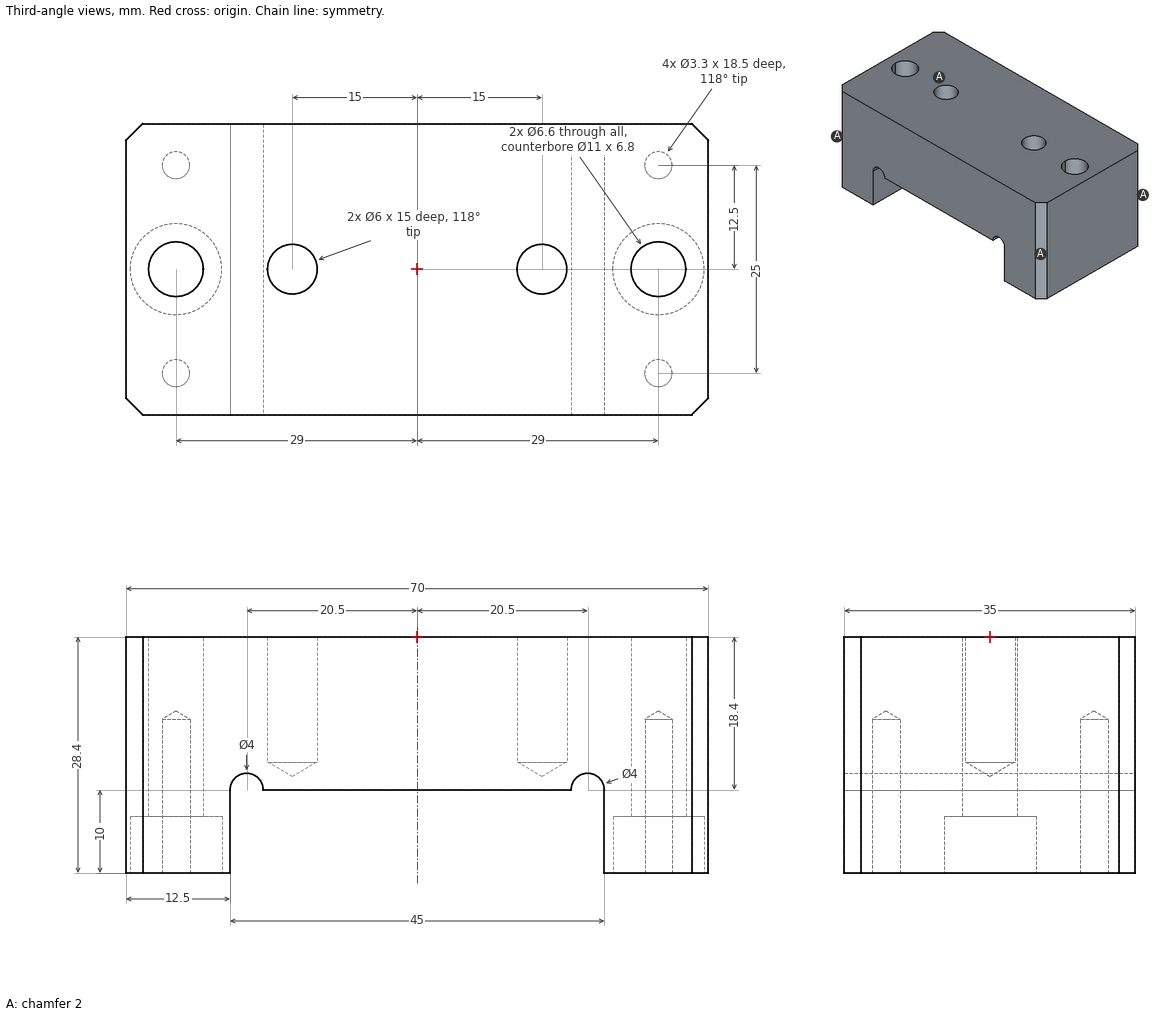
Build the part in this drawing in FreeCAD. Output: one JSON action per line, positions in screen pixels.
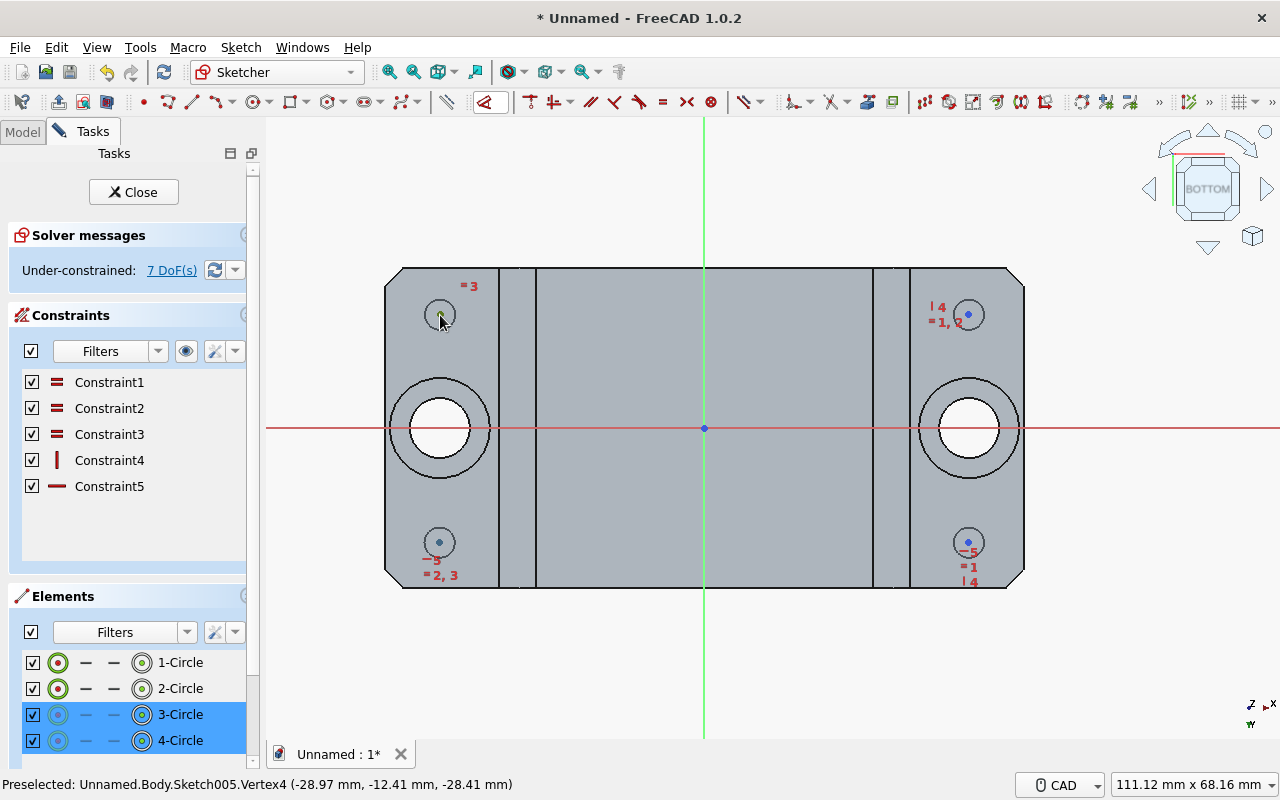
{"action": "left_click", "coordinate": [572, 102]}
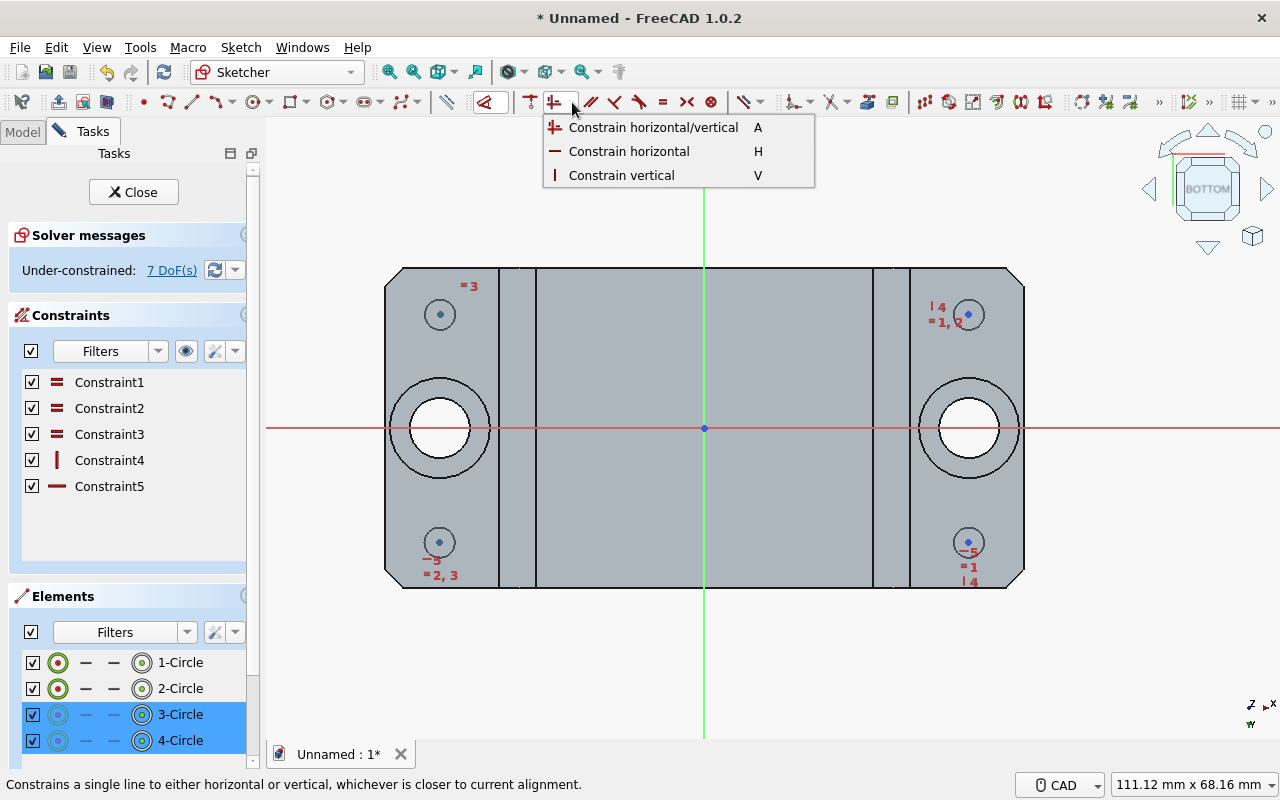
{"action": "left_click", "coordinate": [679, 175]}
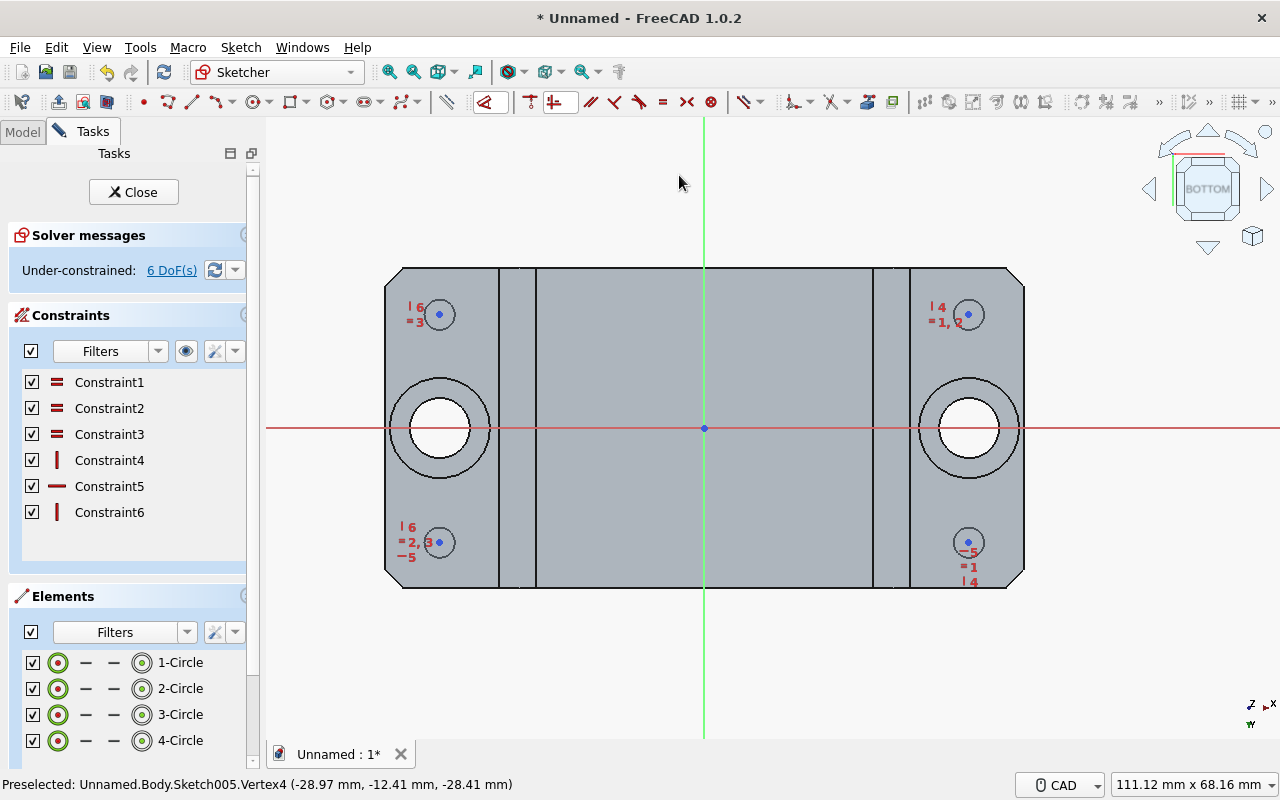
{"action": "left_click", "coordinate": [969, 315]}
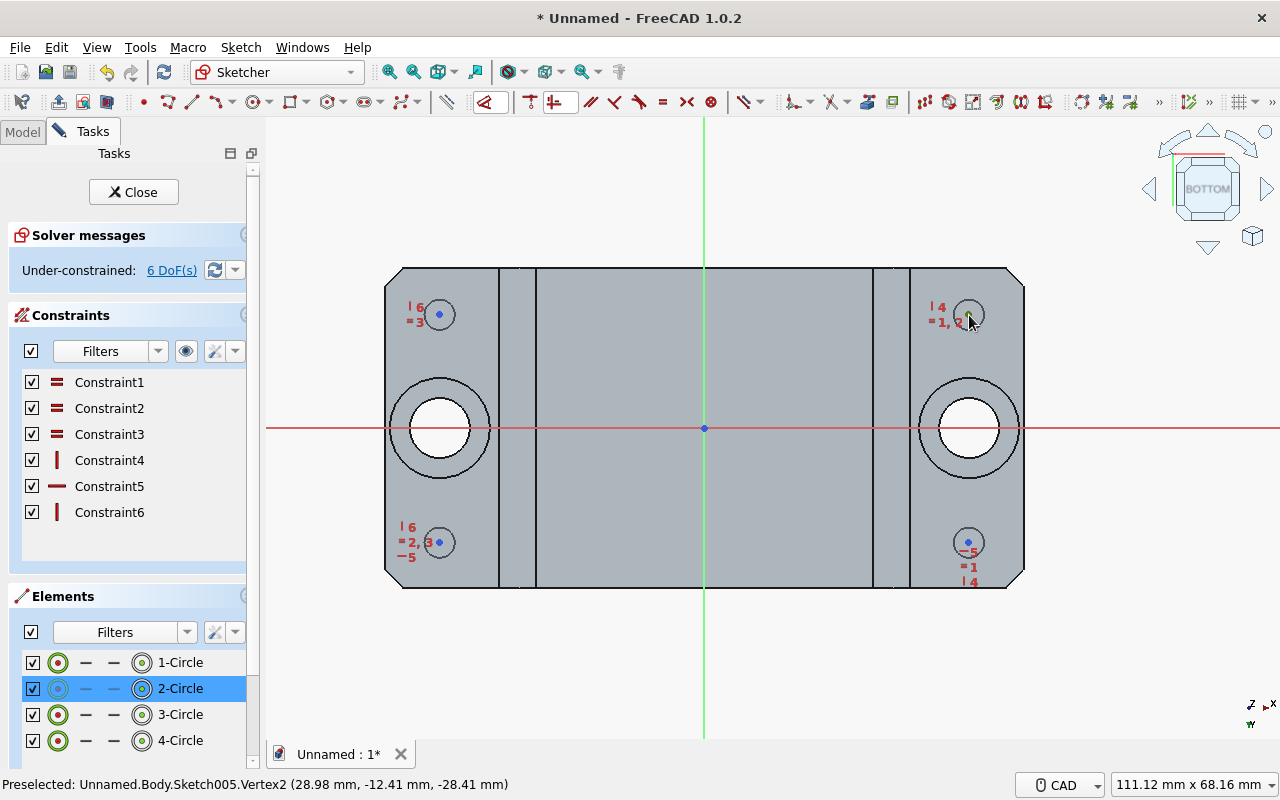
{"action": "left_click", "coordinate": [440, 315]}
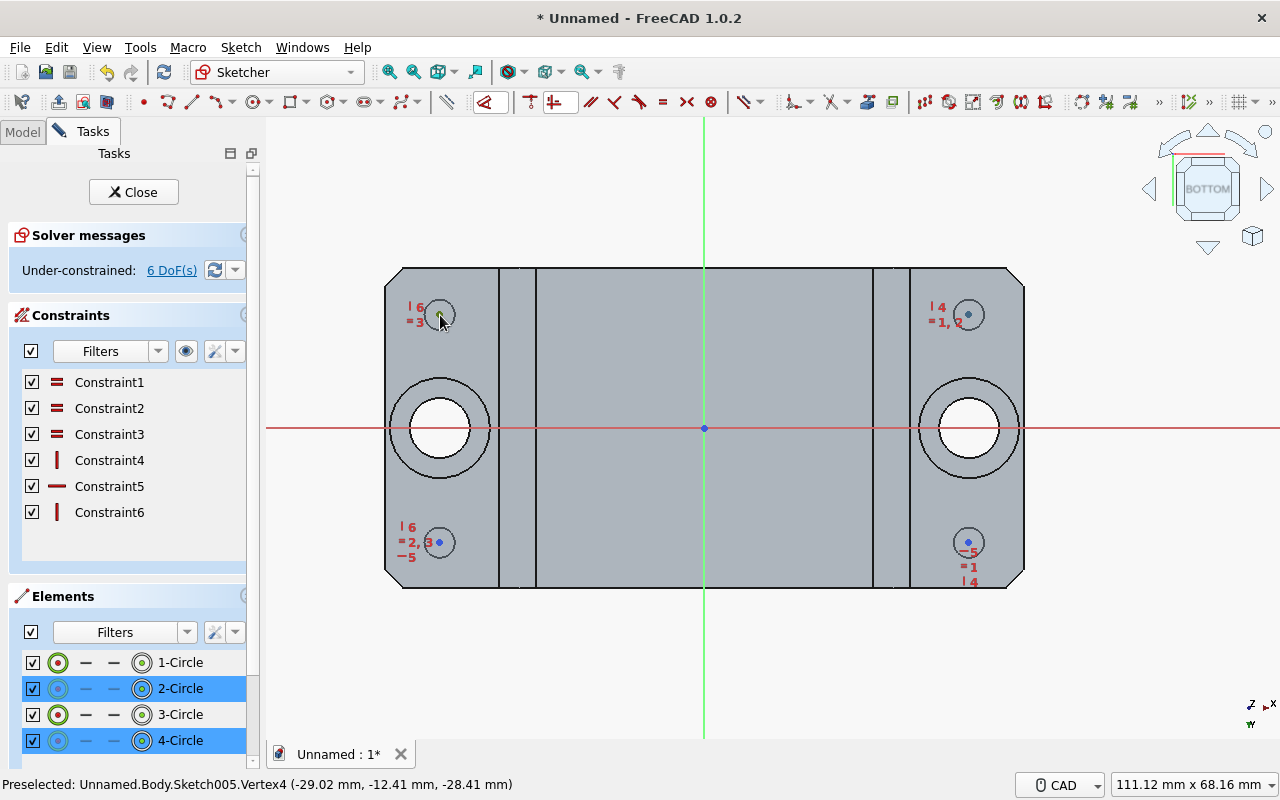
{"action": "key", "text": "h"}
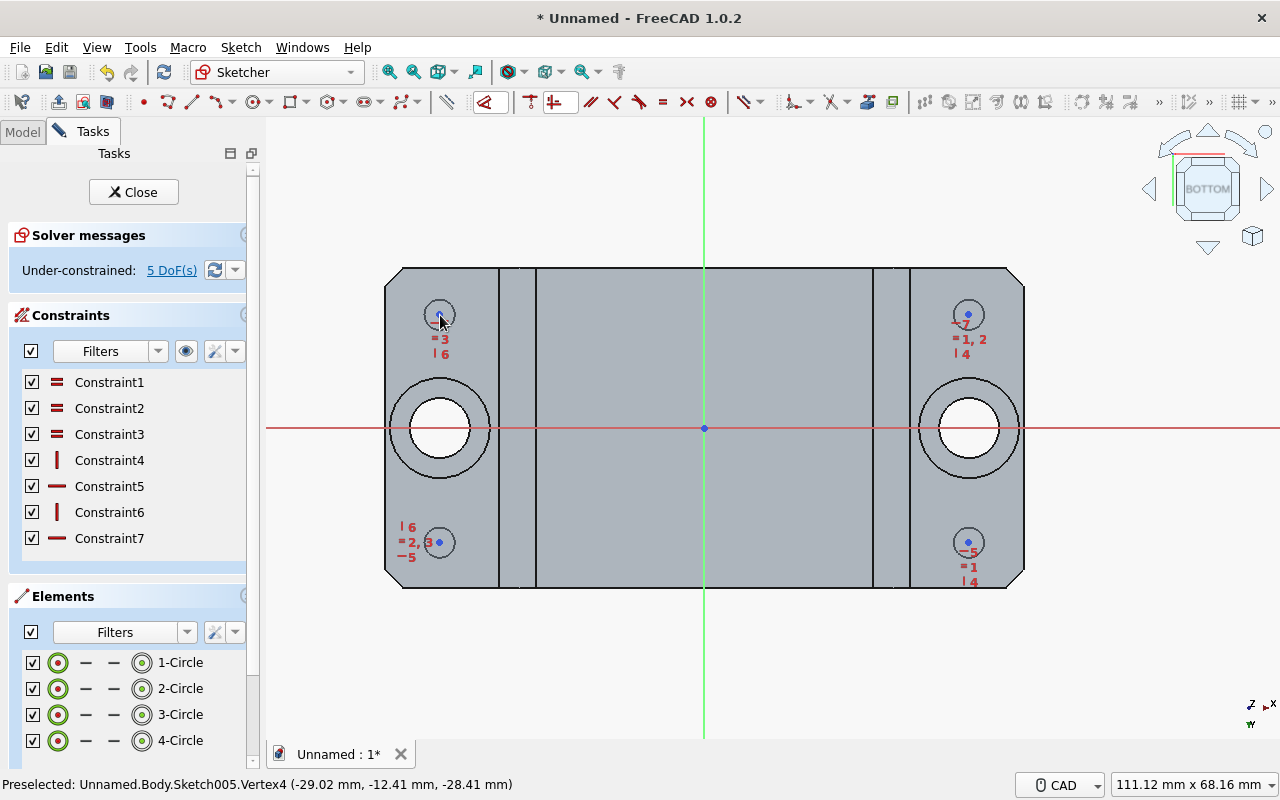
{"action": "key", "text": "d"}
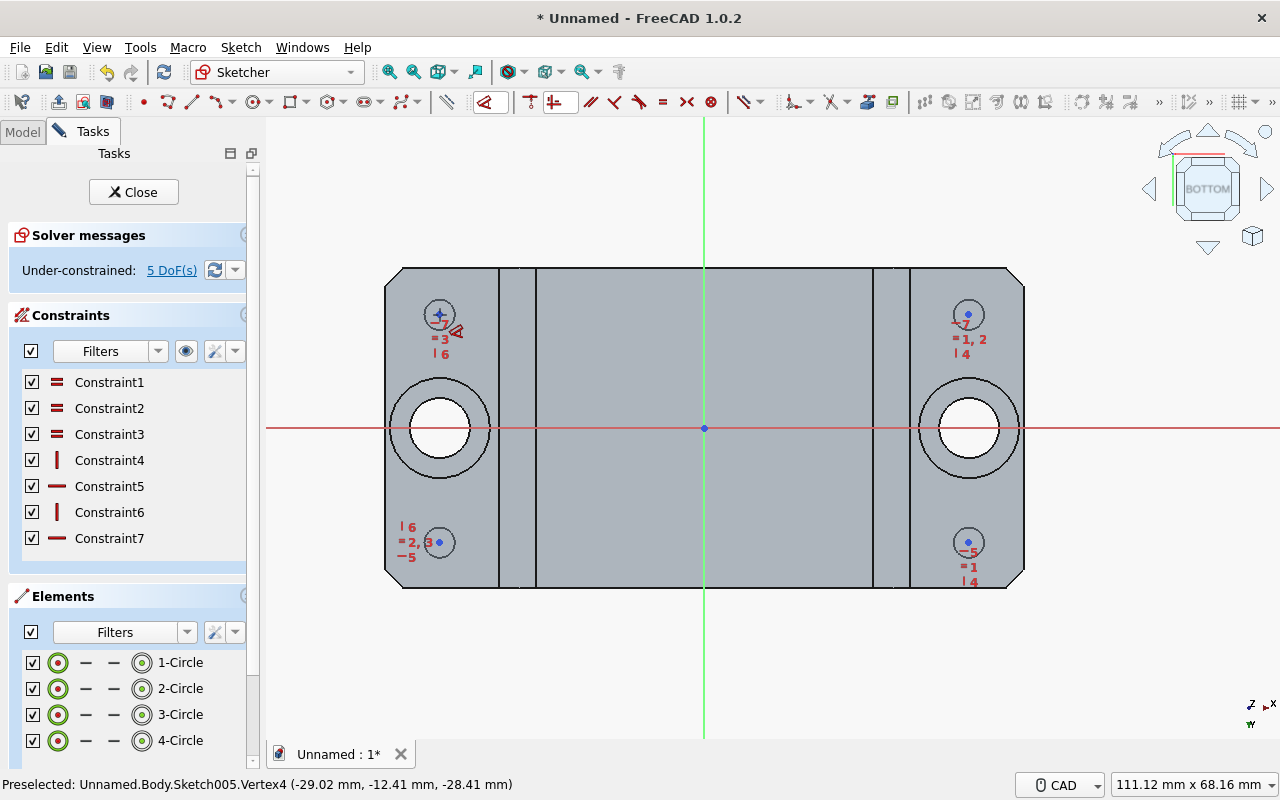
{"action": "scroll", "coordinate": [980, 532], "scroll_direction": "up", "scroll_amount": 2}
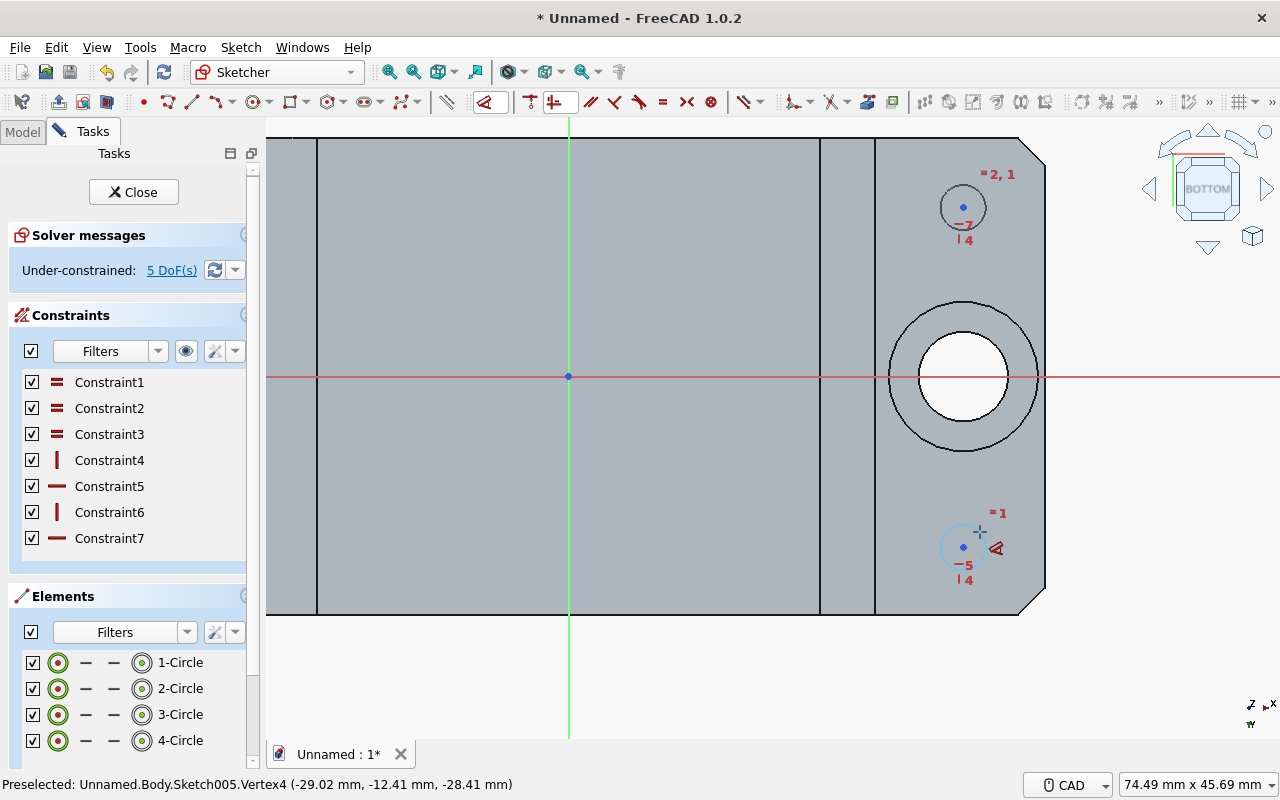
{"action": "left_click", "coordinate": [979, 532]}
{"action": "left_click", "coordinate": [1002, 510]}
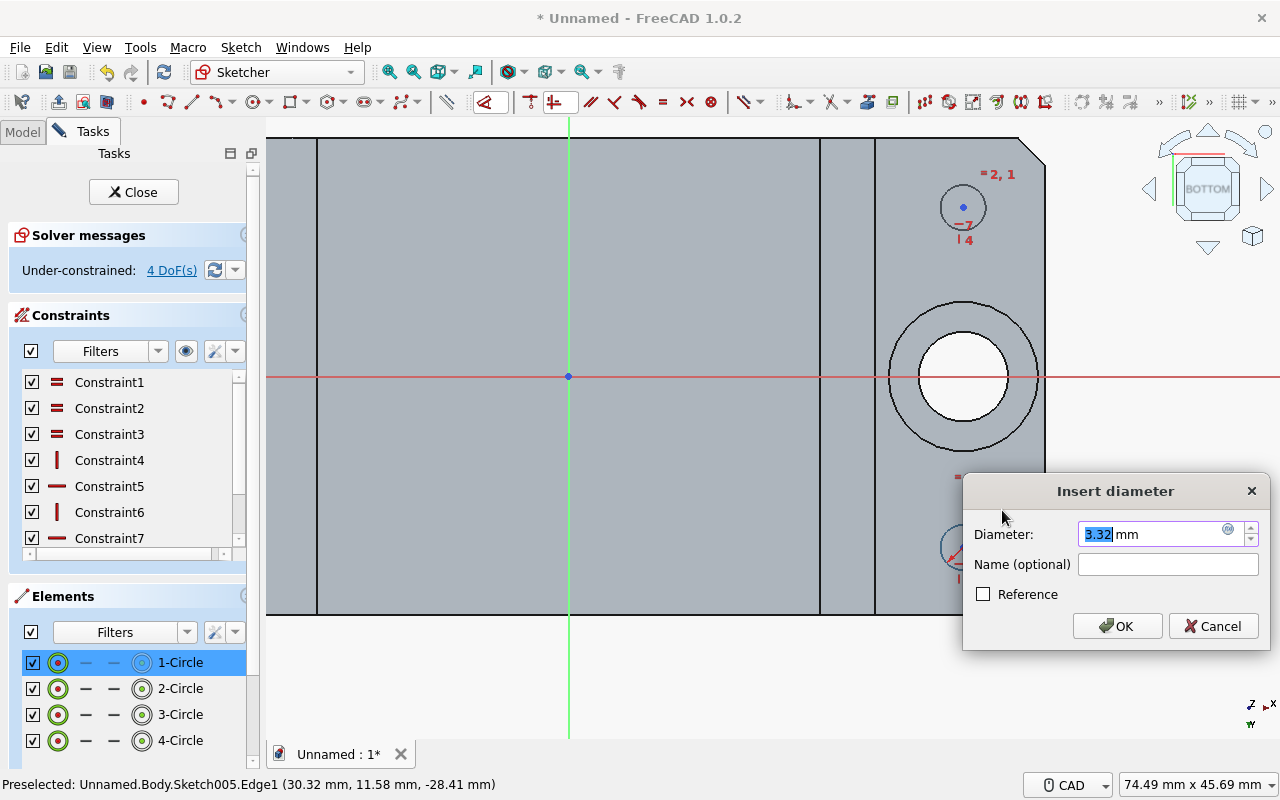
{"action": "type", "text": "3.3"}
{"action": "key", "text": "Return"}